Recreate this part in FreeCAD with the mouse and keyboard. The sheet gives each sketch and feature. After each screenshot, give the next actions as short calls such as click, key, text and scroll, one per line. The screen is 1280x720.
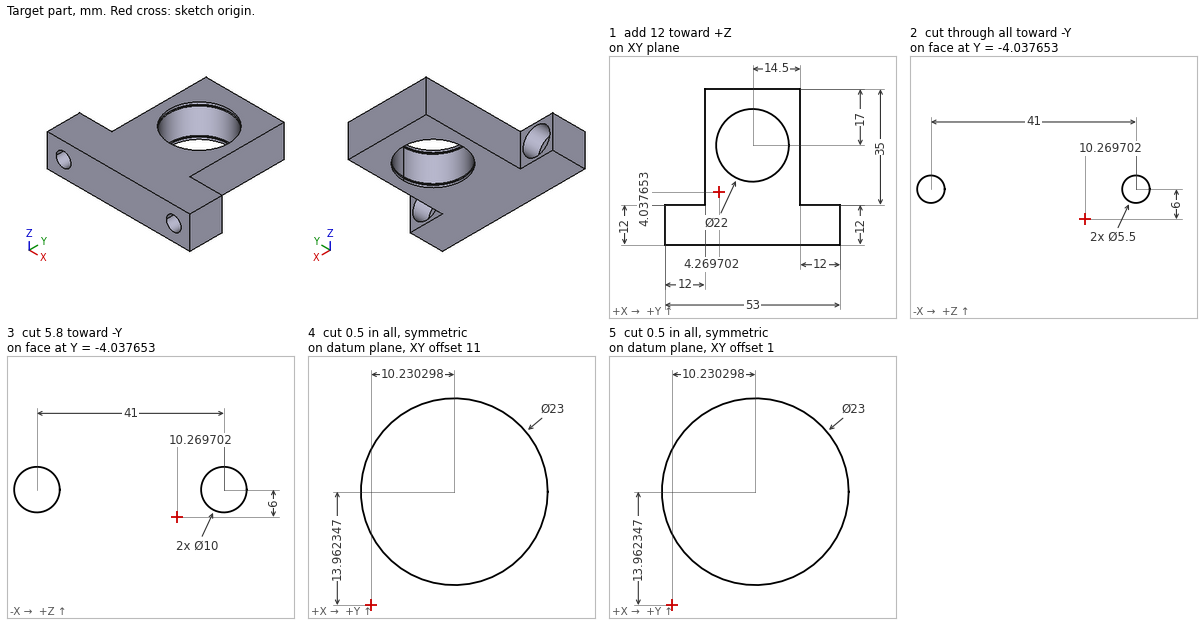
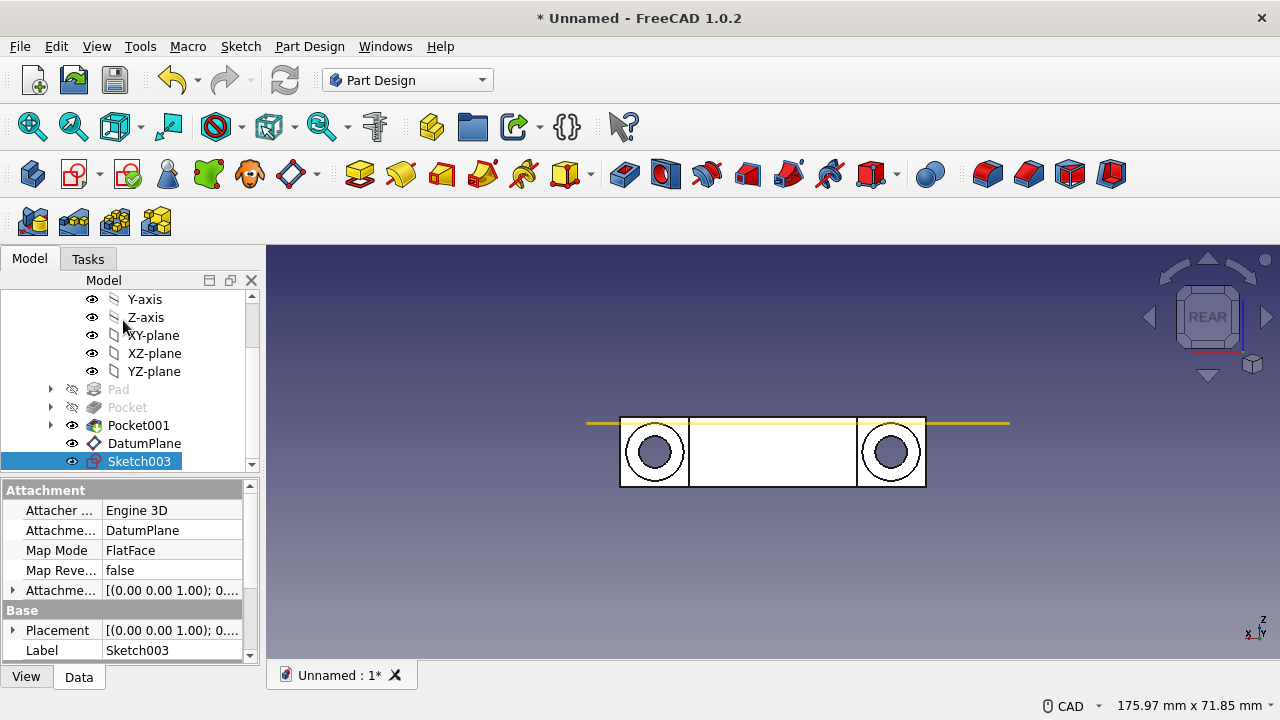
click(625, 174)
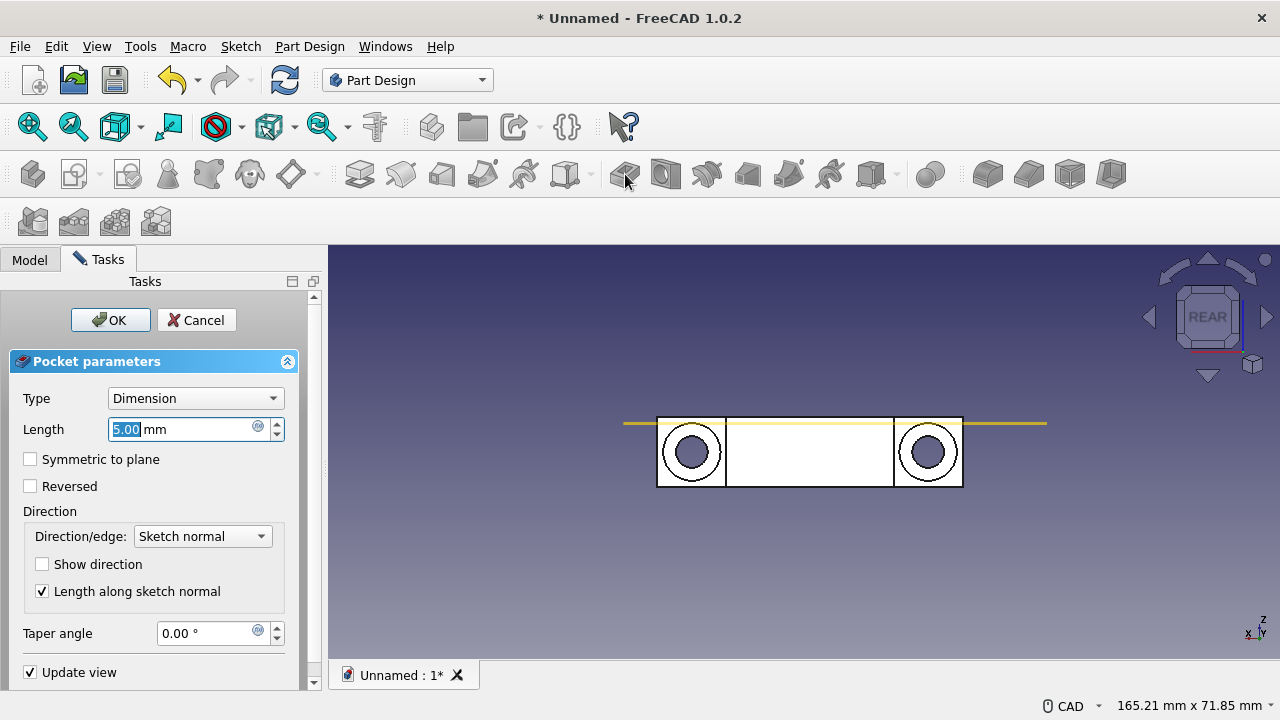
text(0.5)
key(Tab)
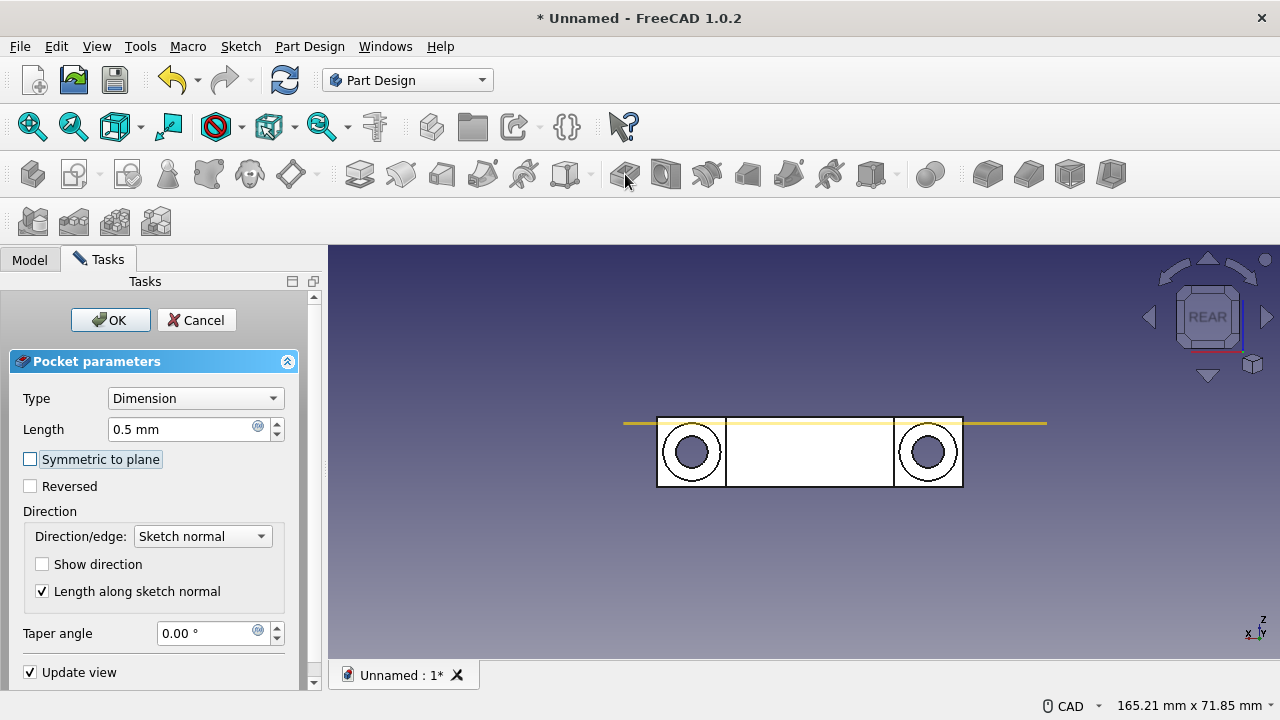
click(31, 459)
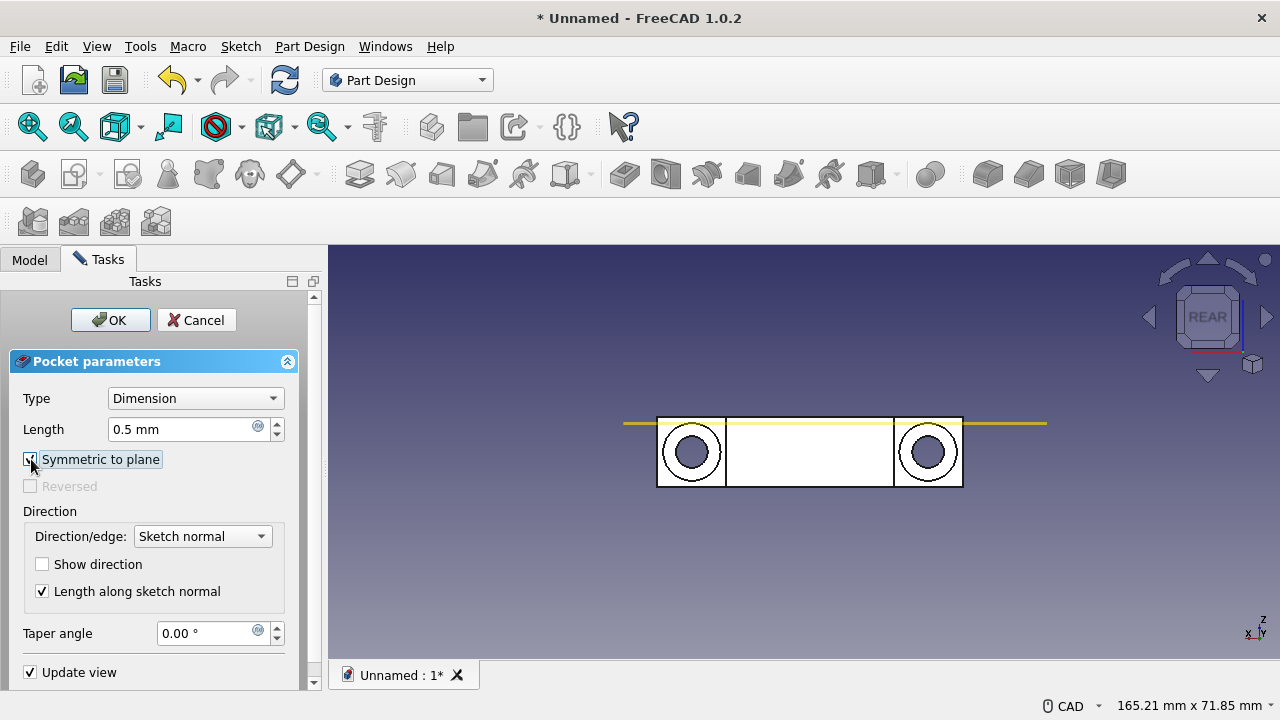
click(111, 320)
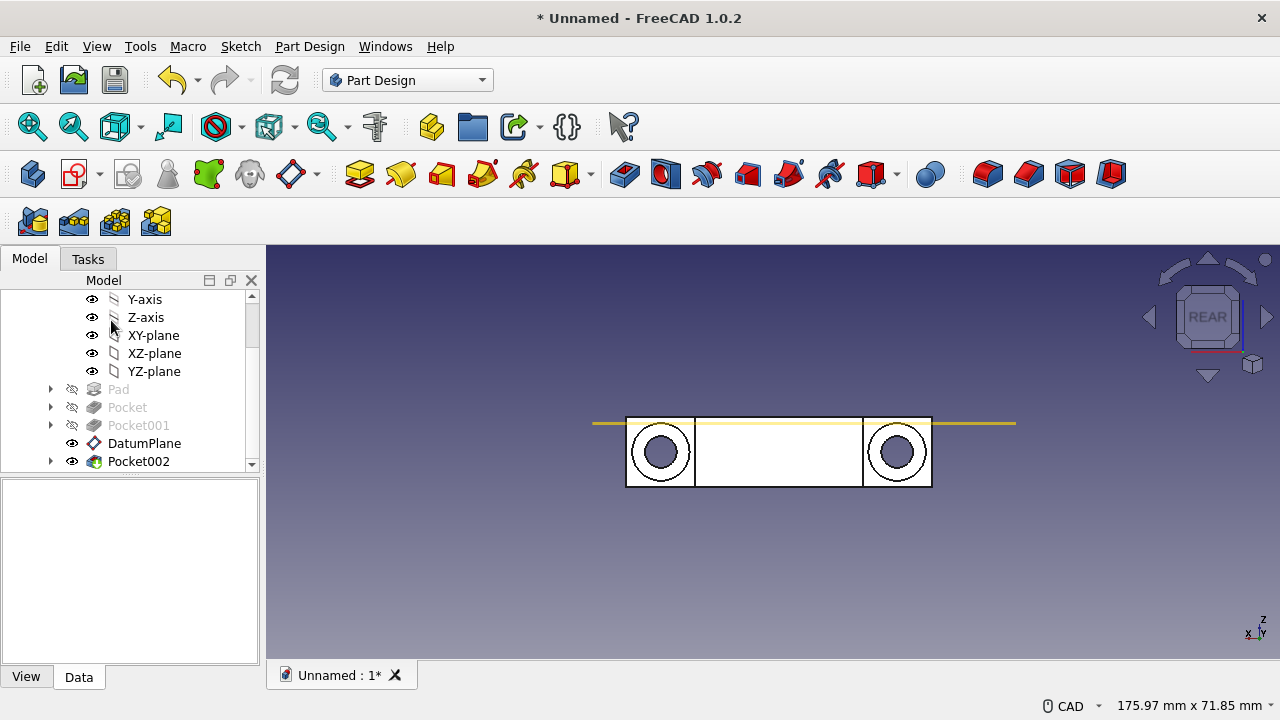
click(117, 443)
key(space)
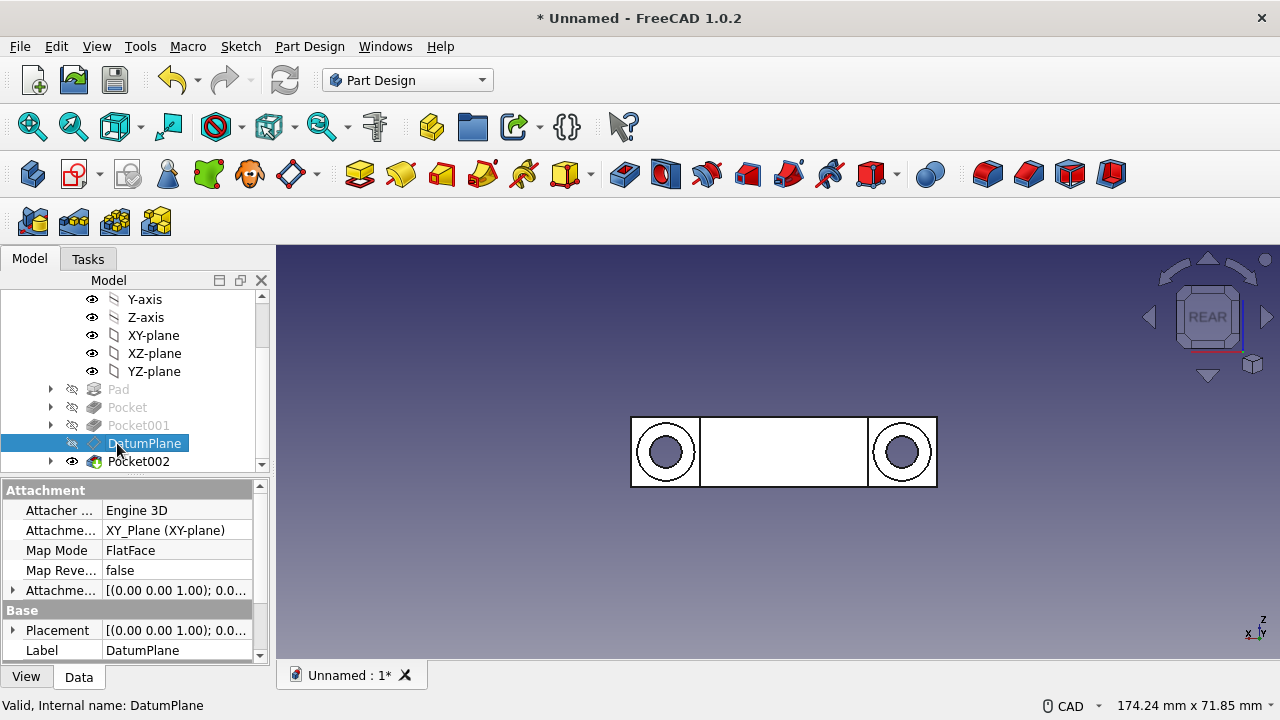
click(33, 128)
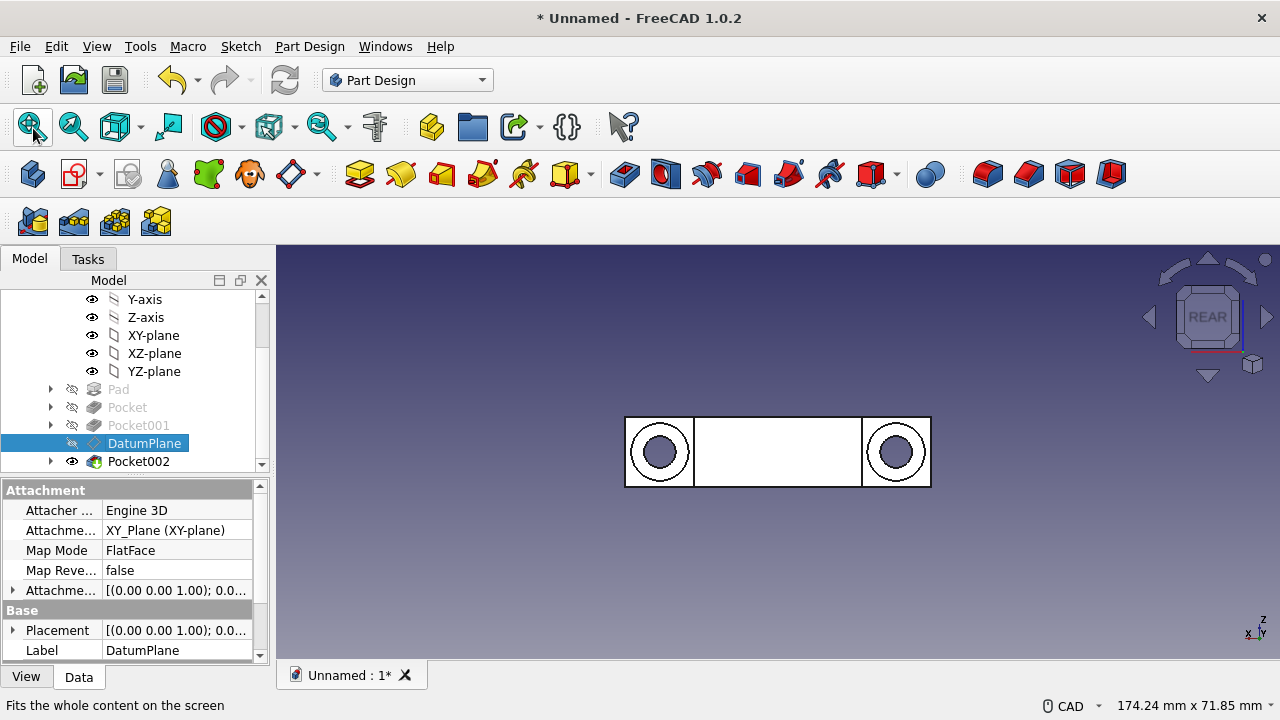
scroll(161, 385, down, 3)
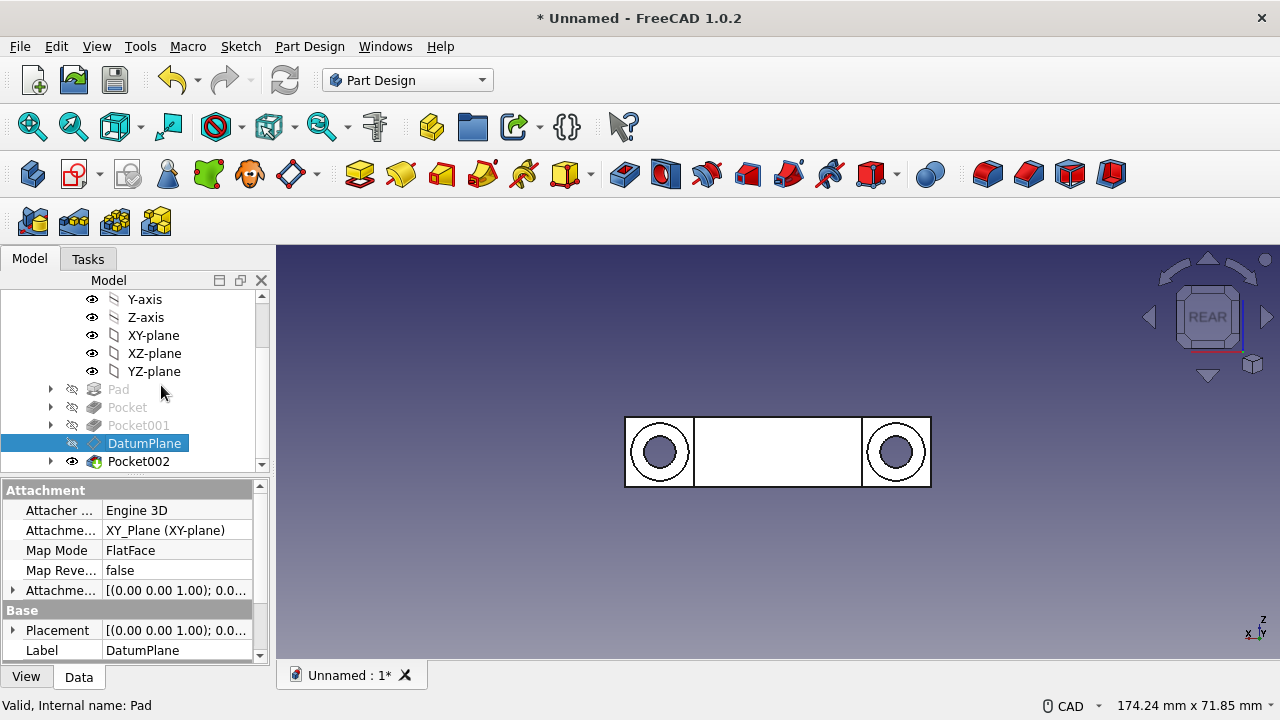
scroll(161, 385, up, 15)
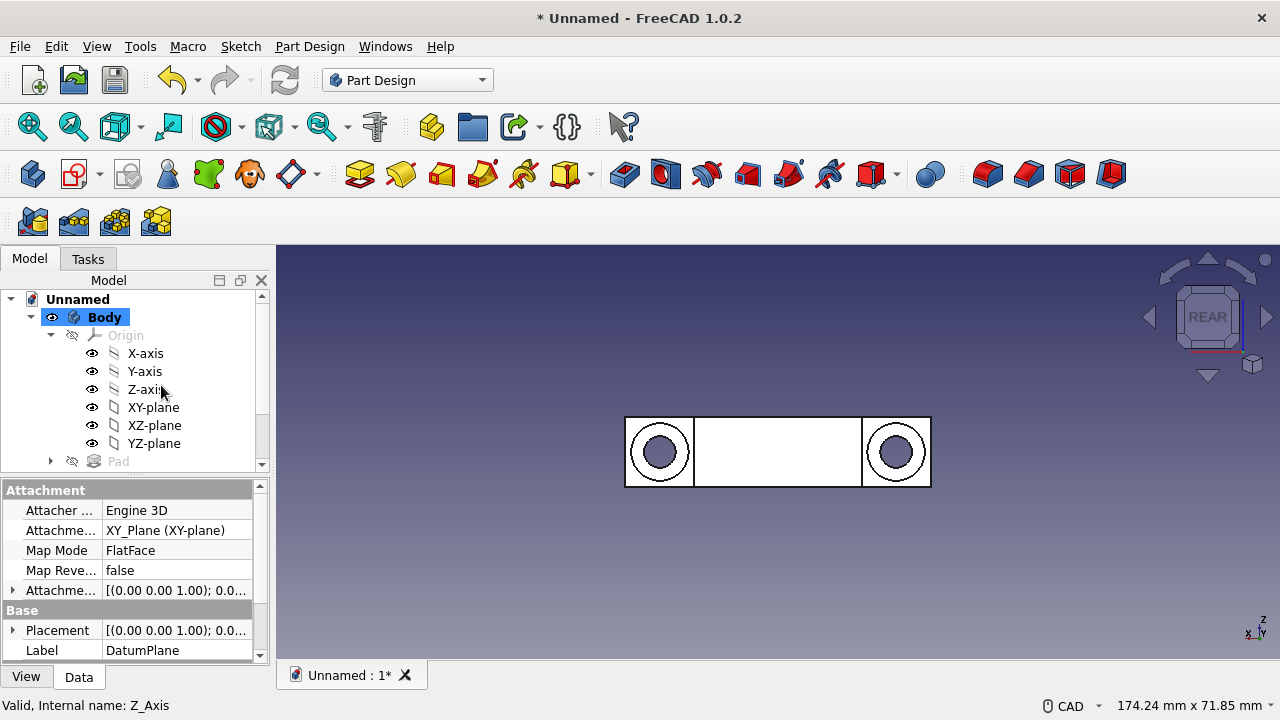
click(137, 407)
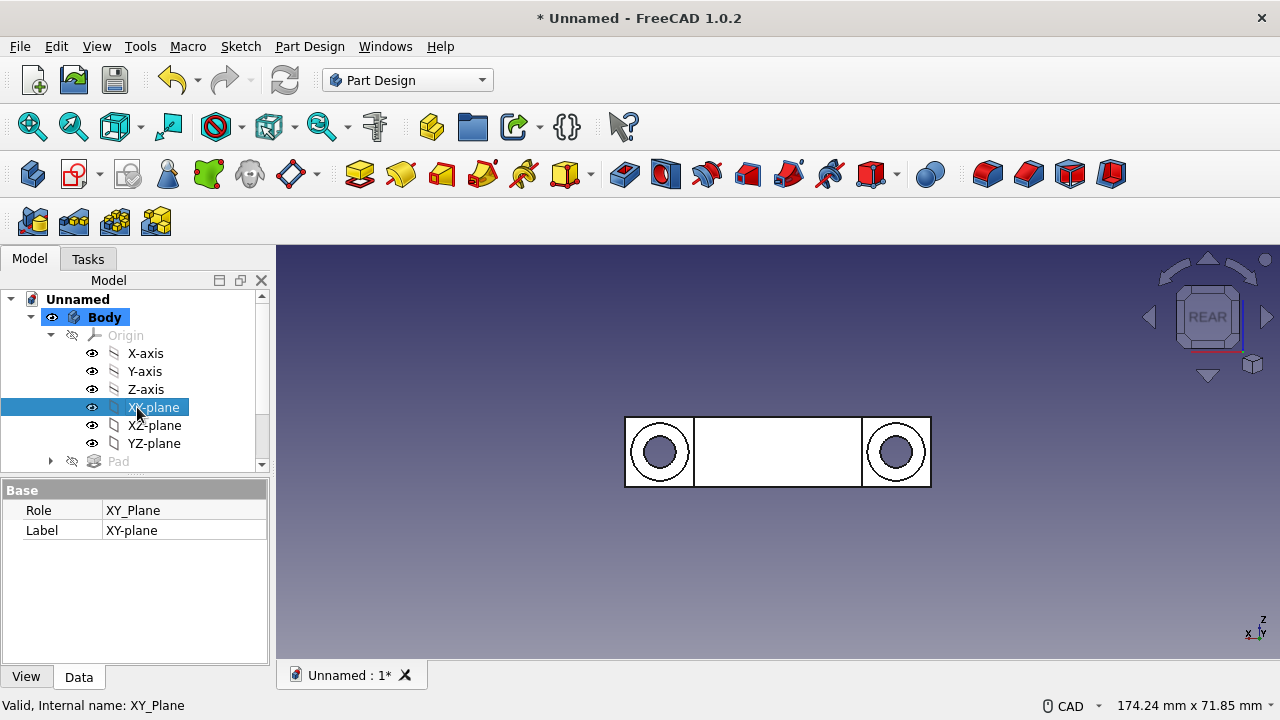
click(290, 174)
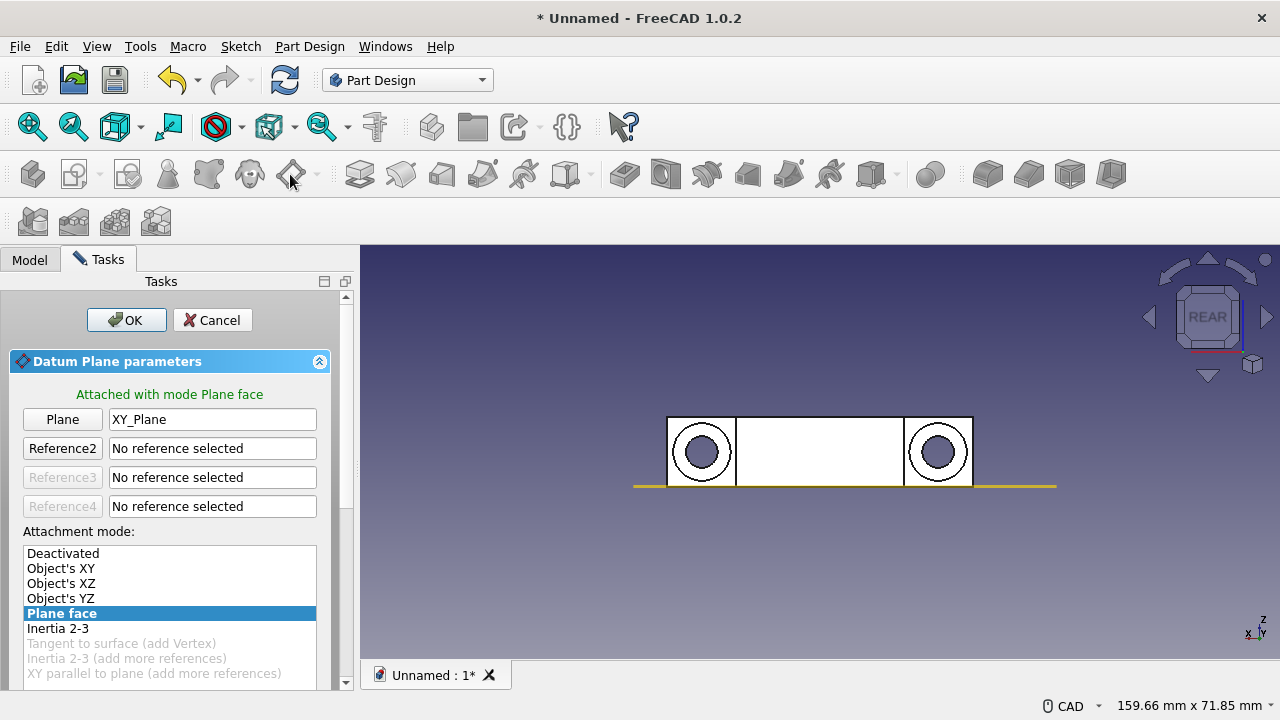
scroll(346, 490, down, 4)